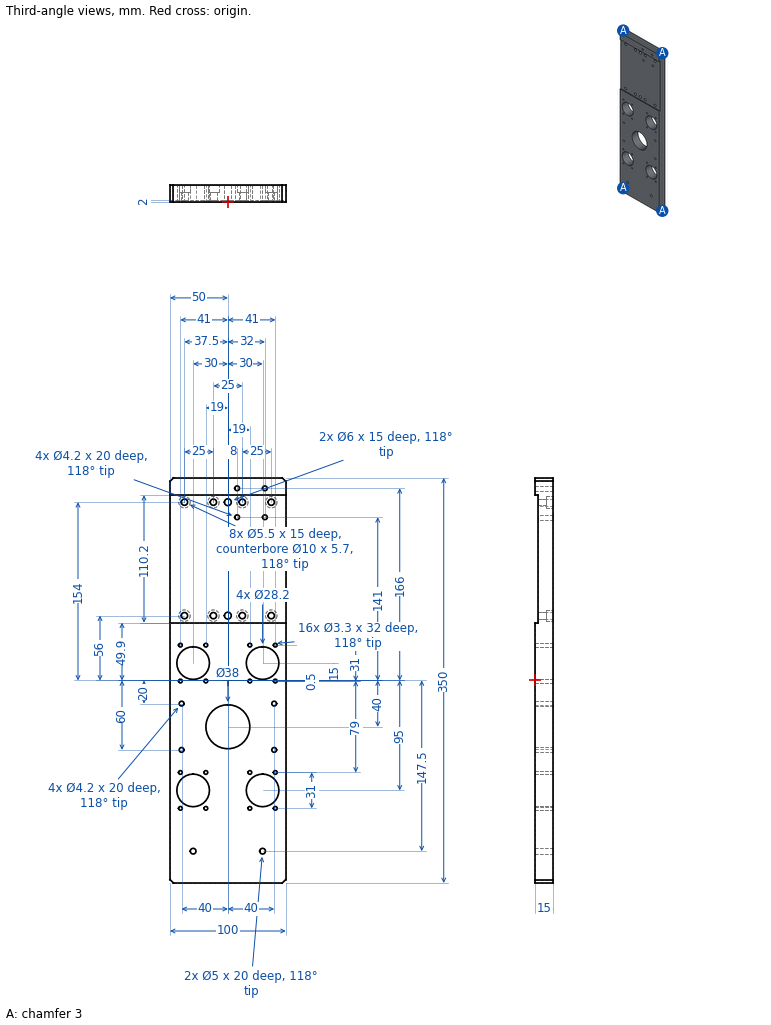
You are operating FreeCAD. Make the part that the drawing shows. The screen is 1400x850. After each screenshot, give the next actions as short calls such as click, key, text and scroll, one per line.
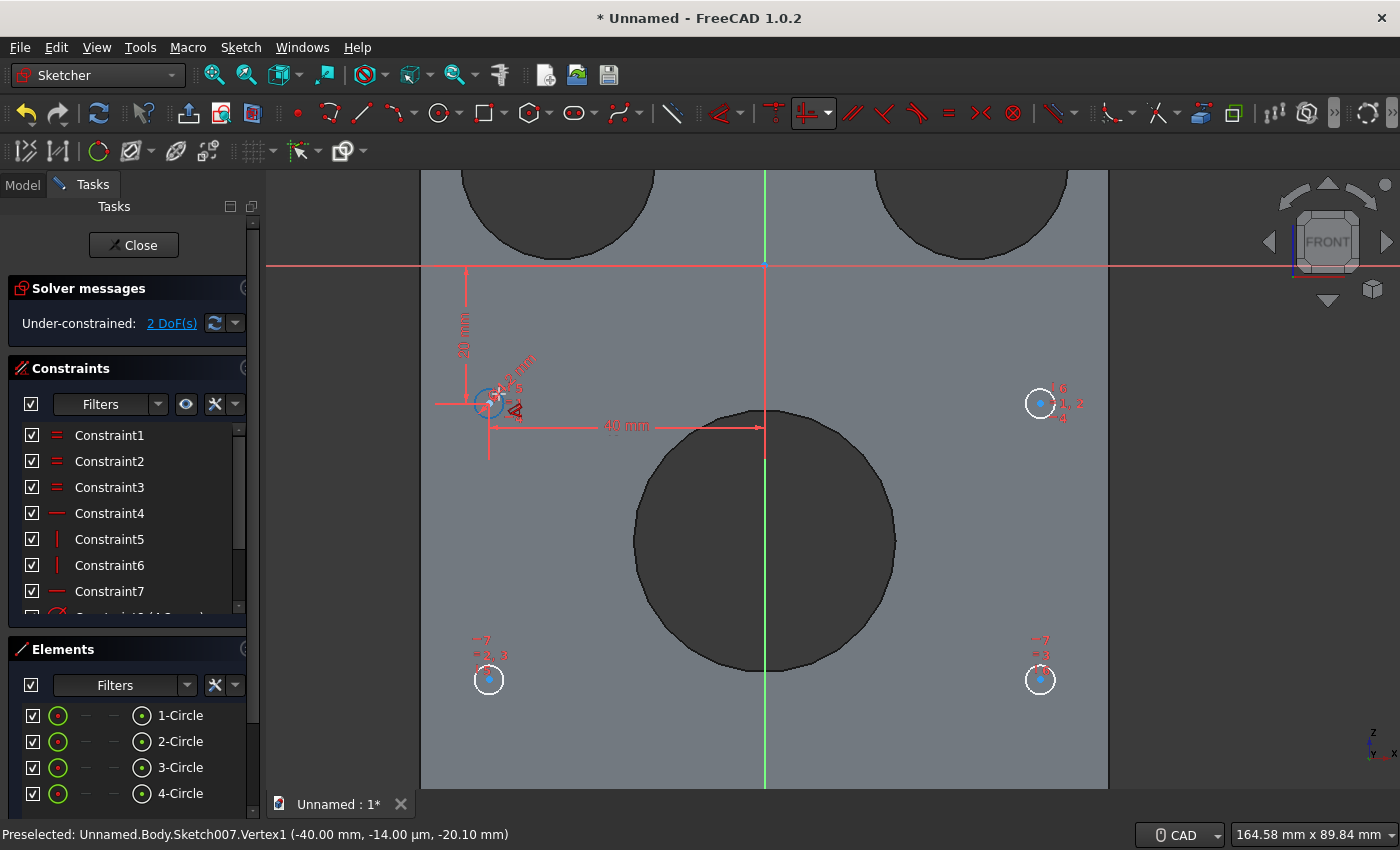
click(1040, 404)
click(902, 232)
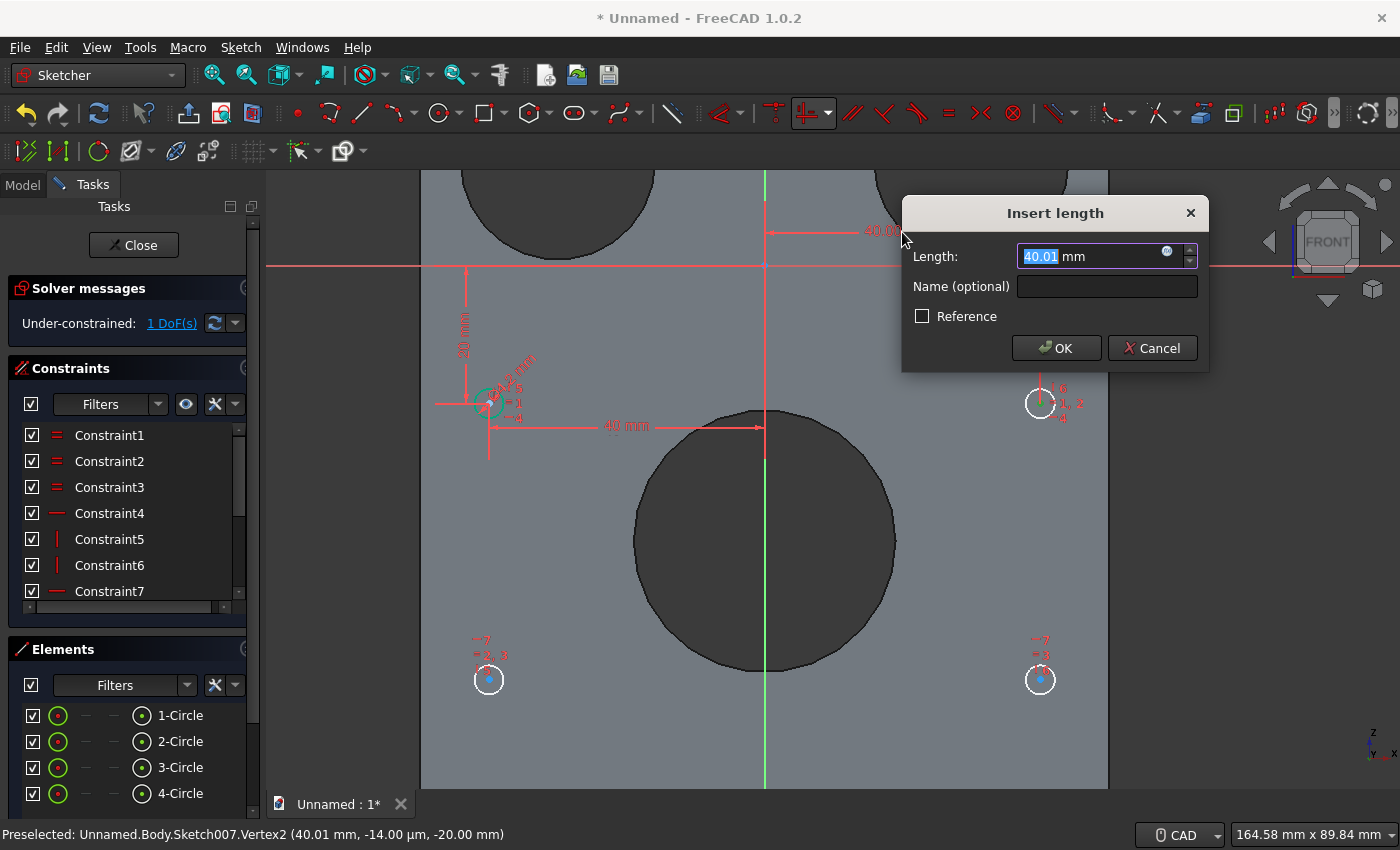
text(40)
key(Return)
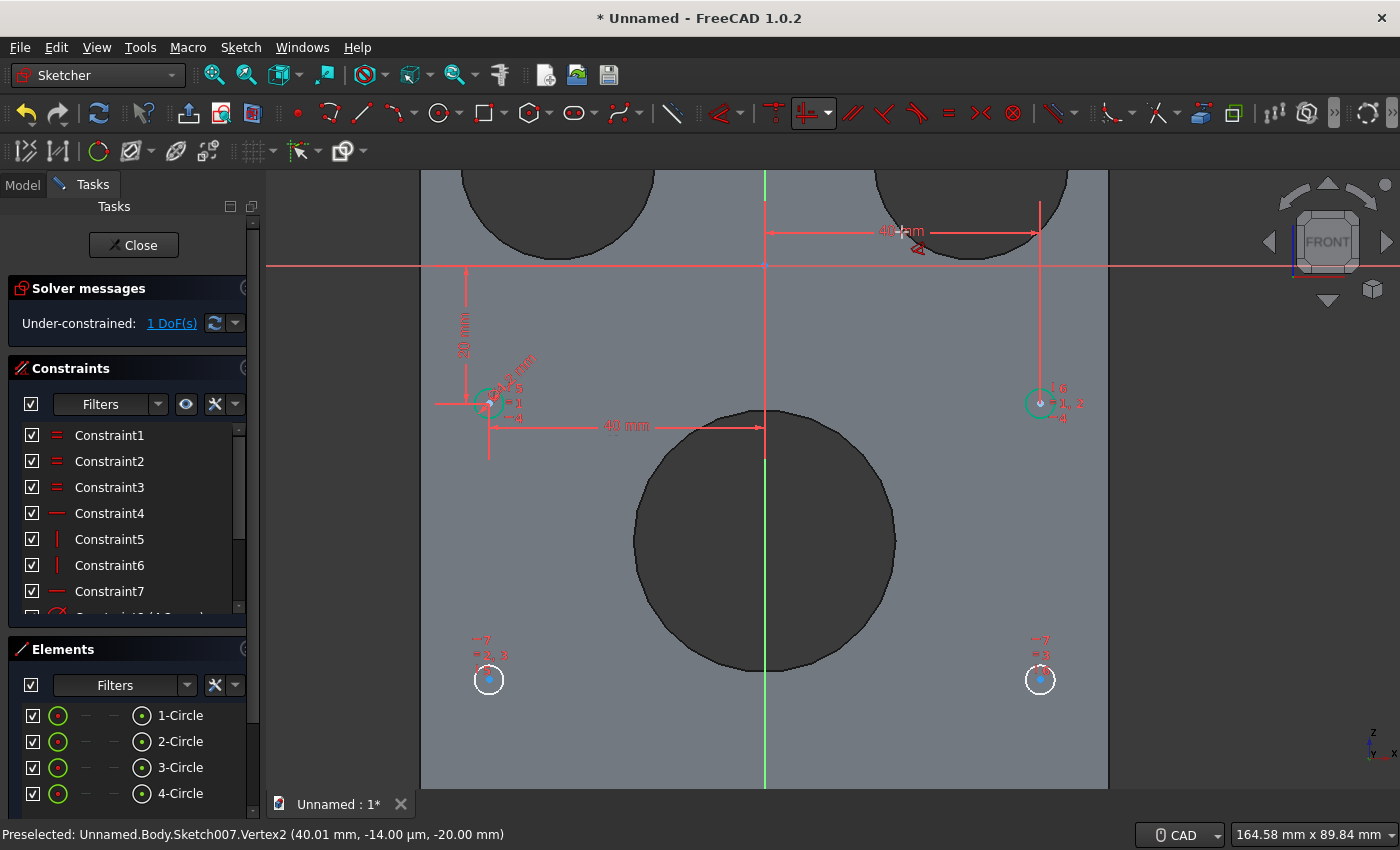
click(489, 680)
click(455, 473)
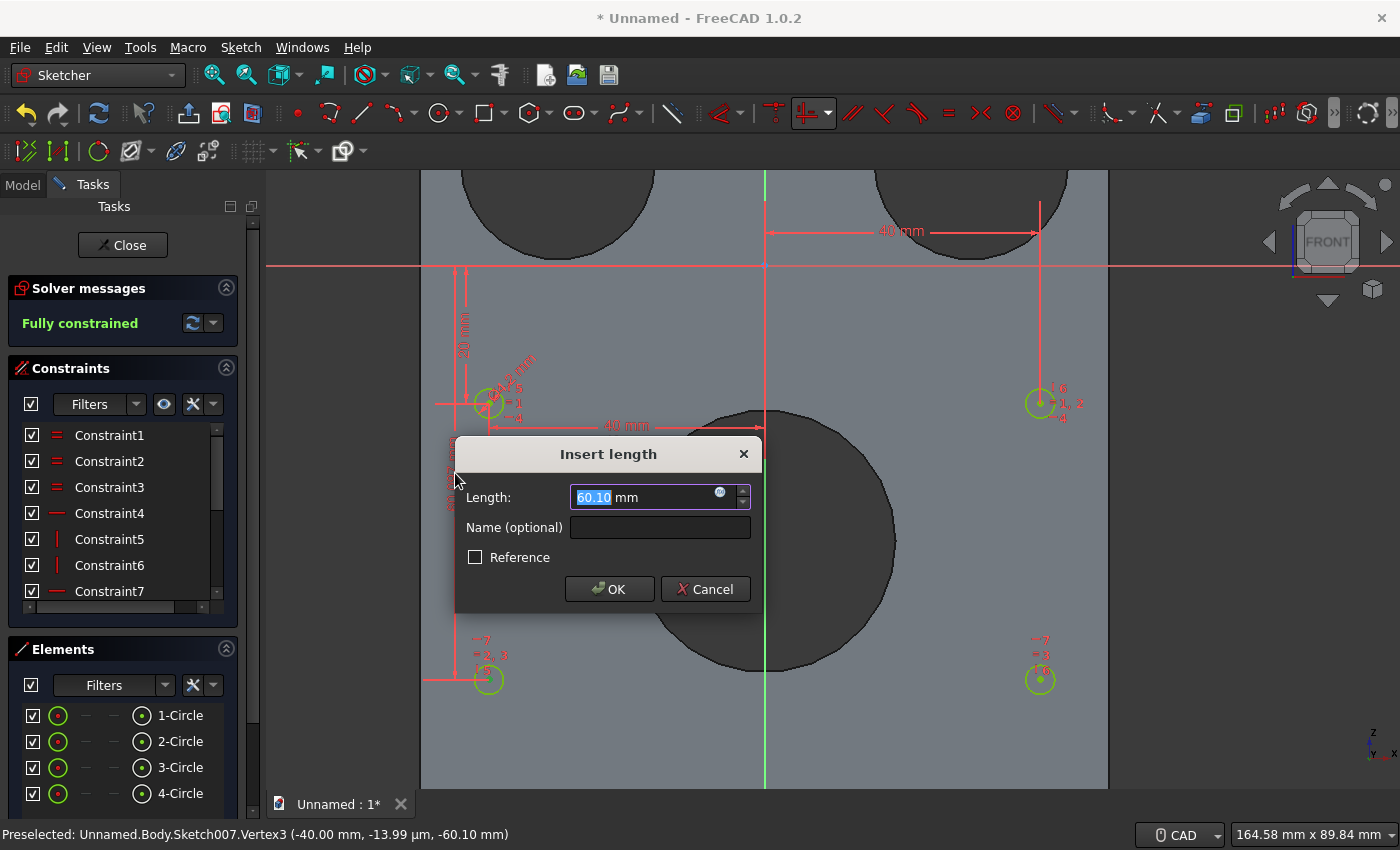
text(60)
key(Return)
key(Escape)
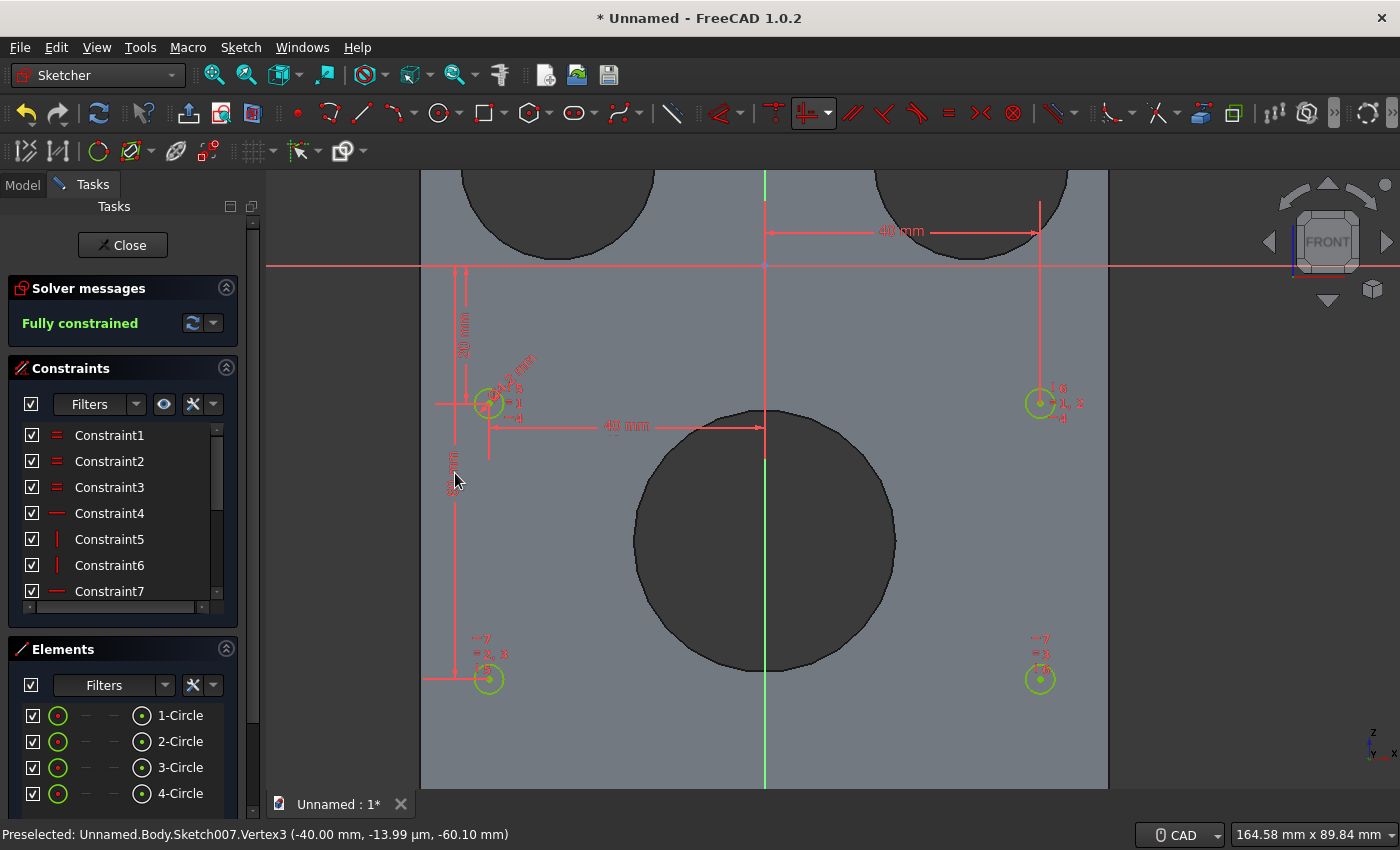
click(123, 245)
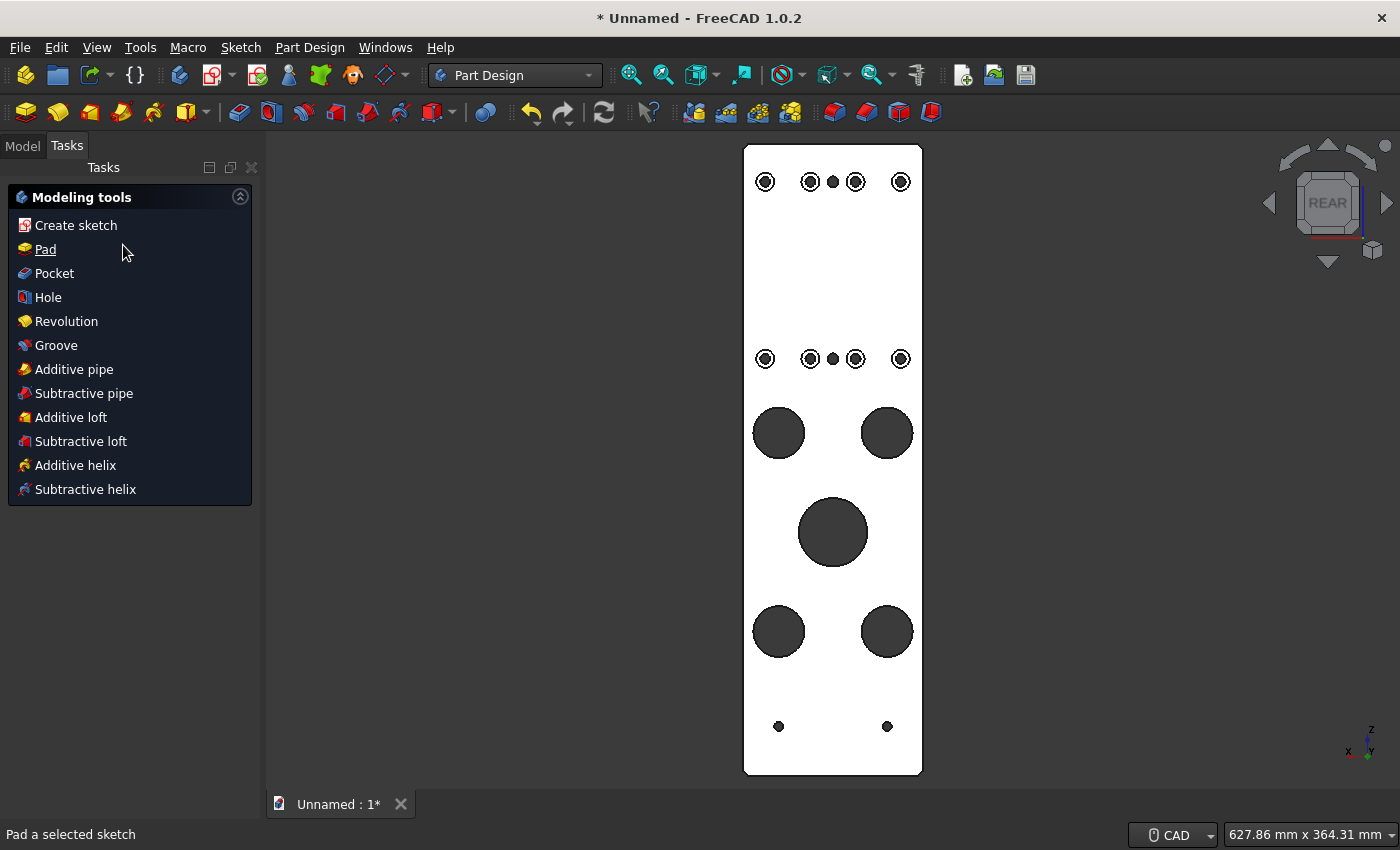
click(272, 112)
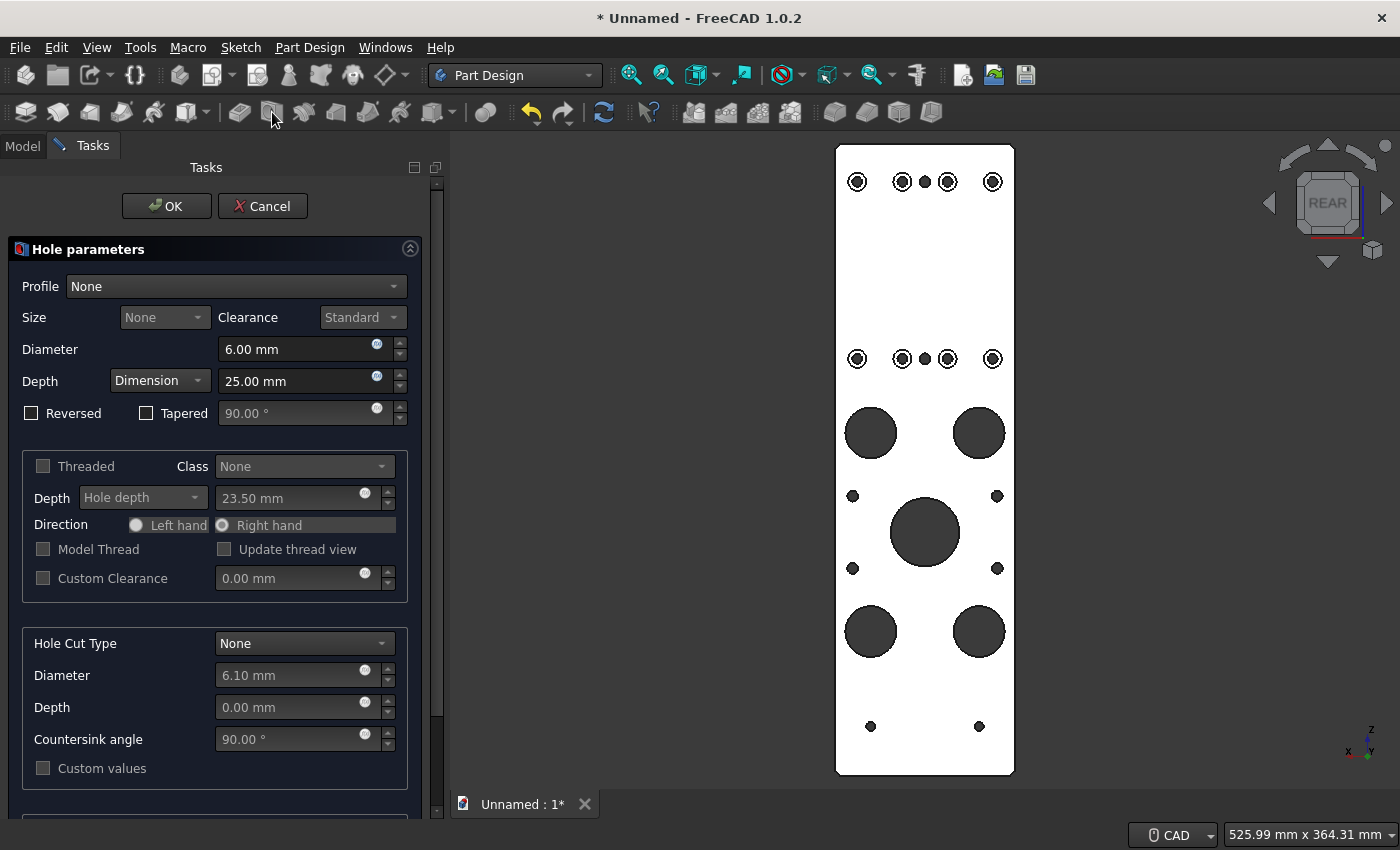
triple_click(305, 349)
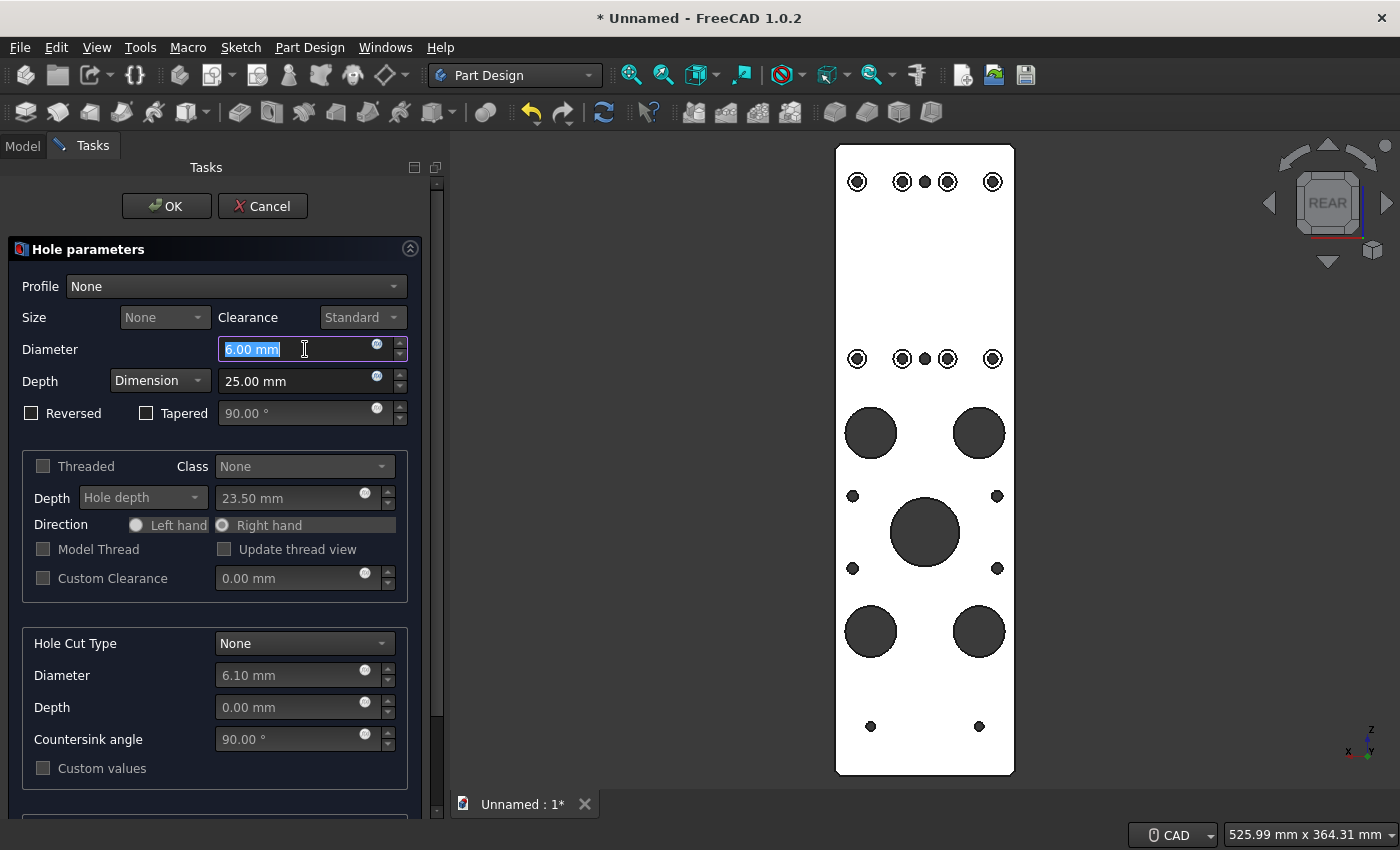
text(4.2)
key(Tab)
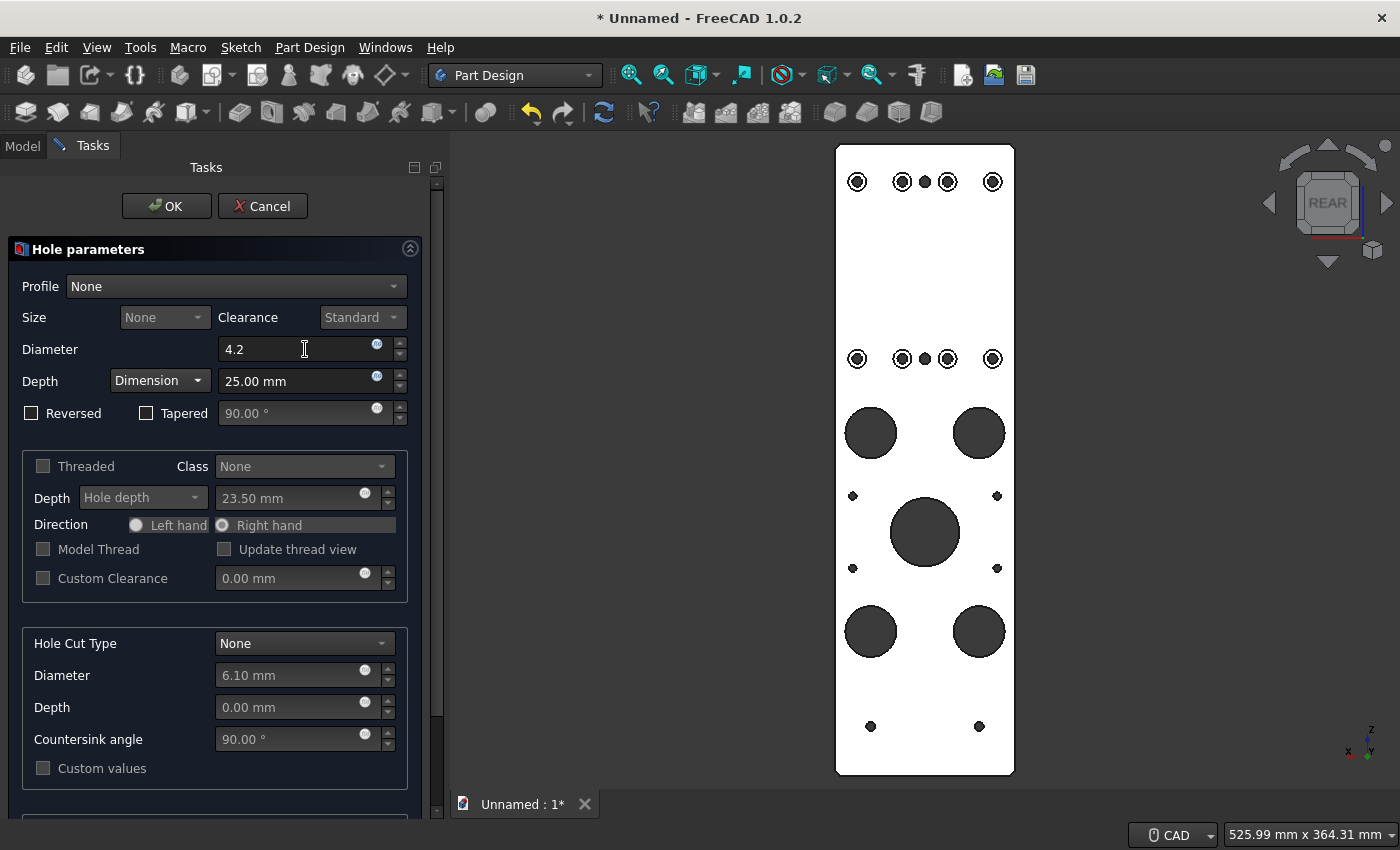
triple_click(305, 381)